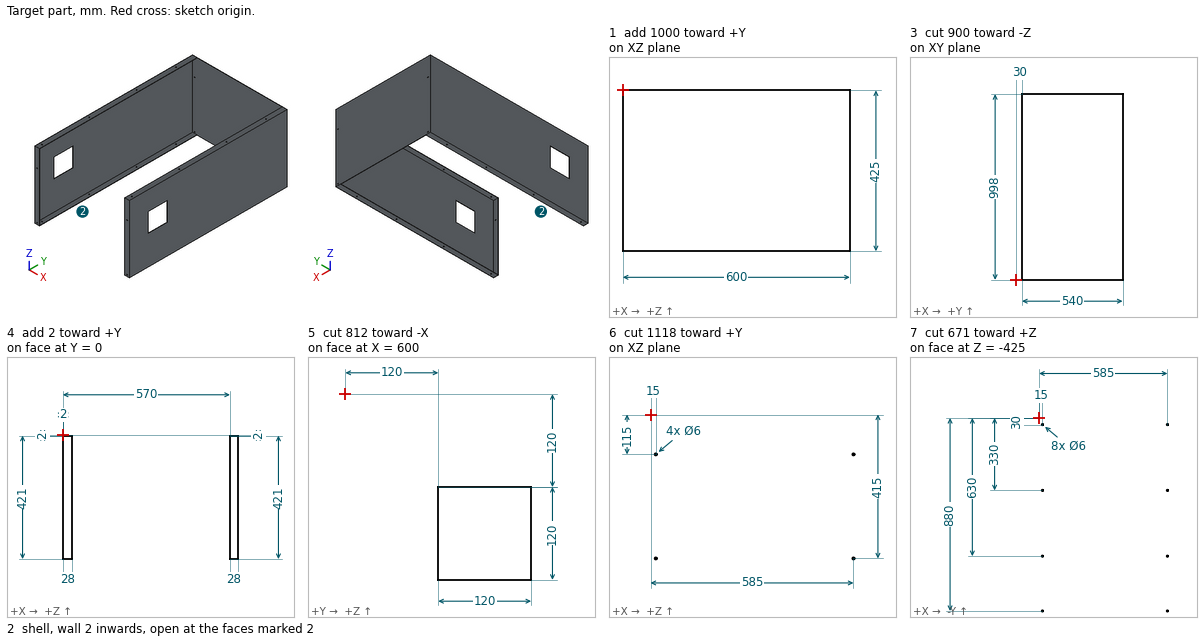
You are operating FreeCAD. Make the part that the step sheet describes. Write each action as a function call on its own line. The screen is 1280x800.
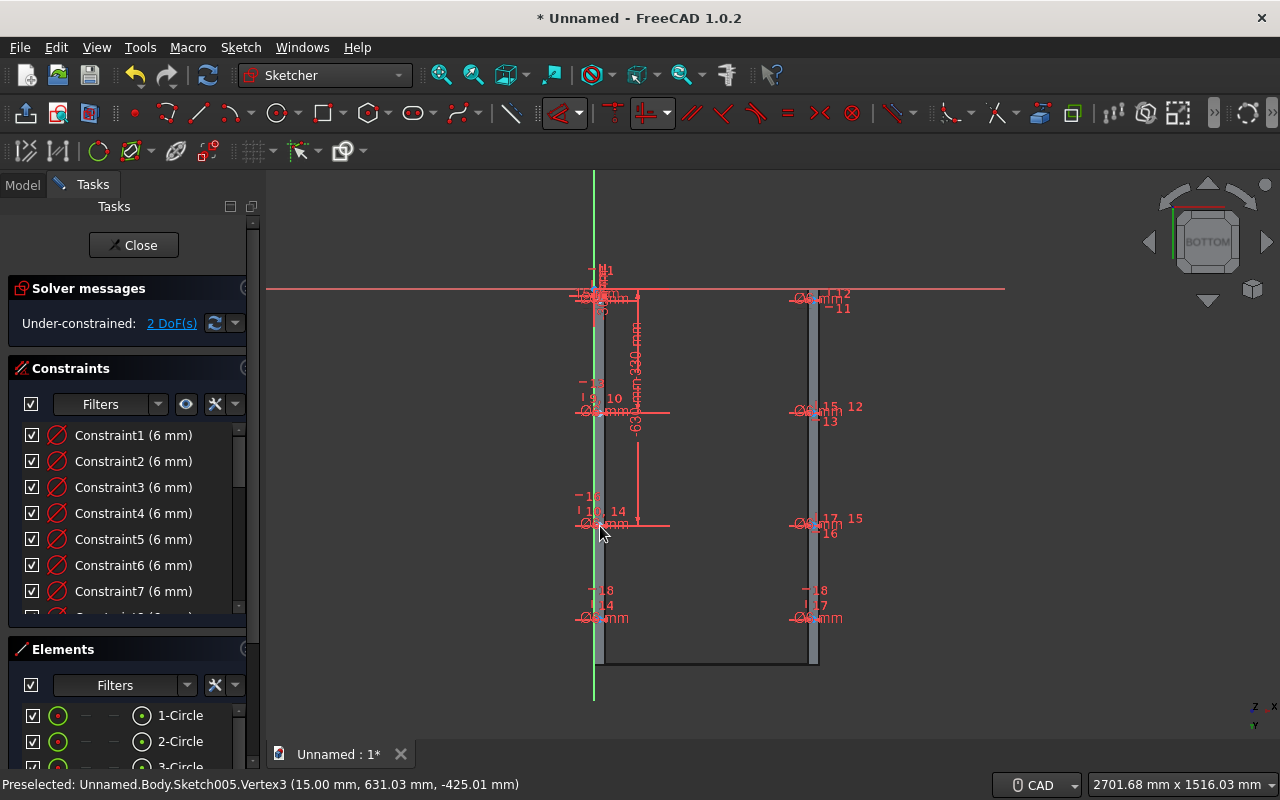
click(814, 301)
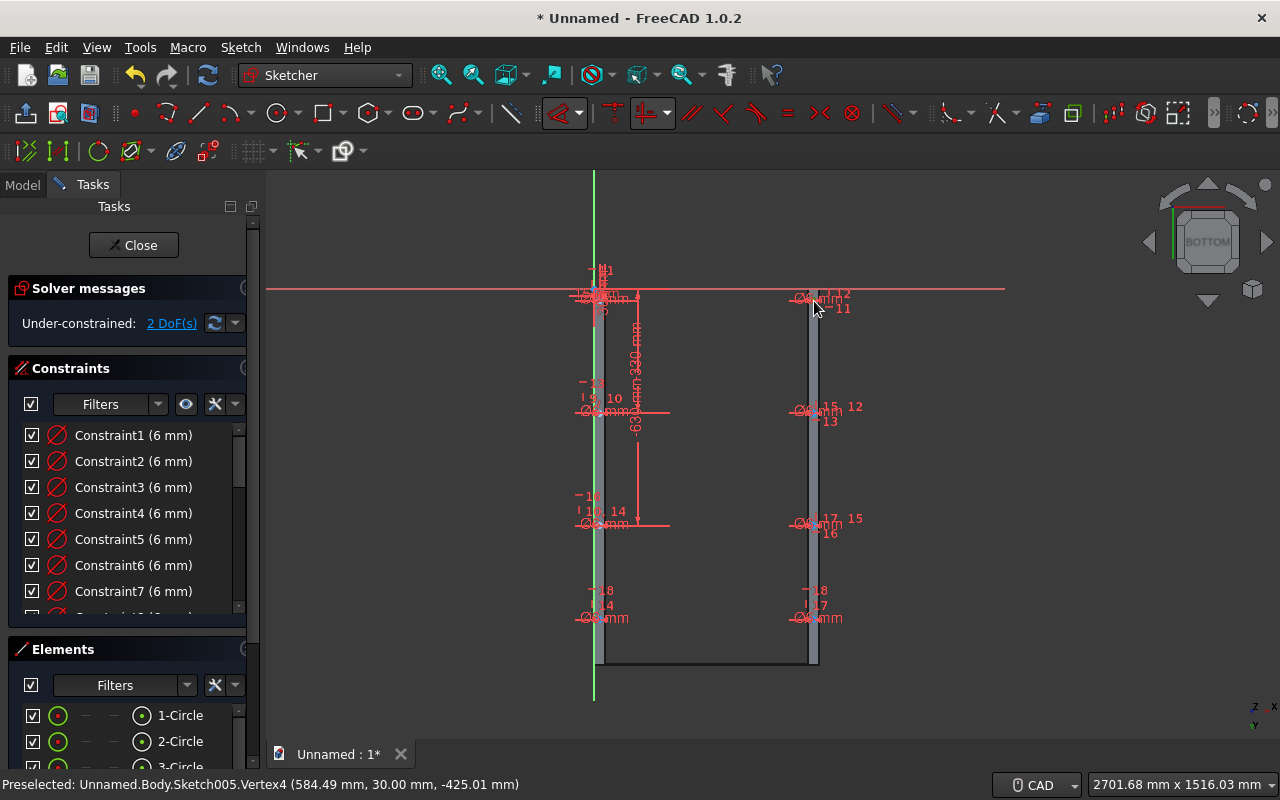
key(l)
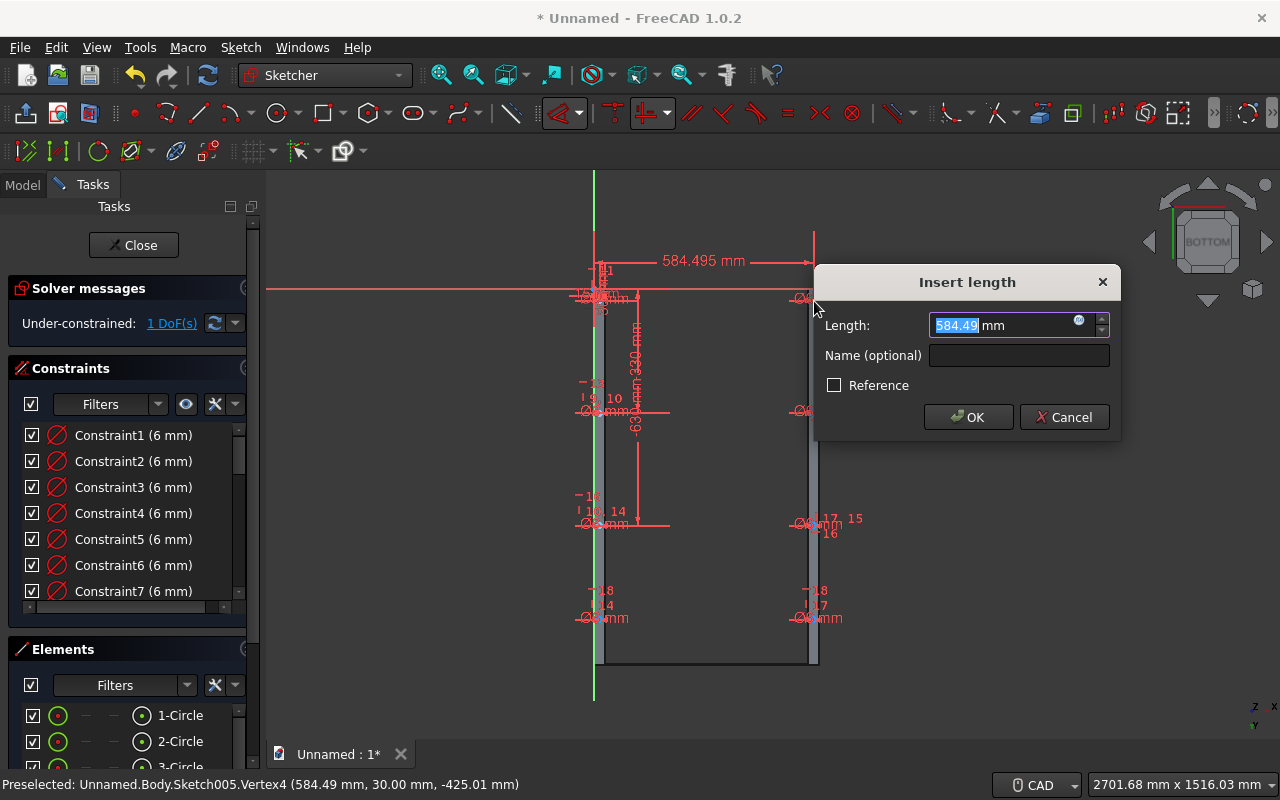
text(585)
key(Return)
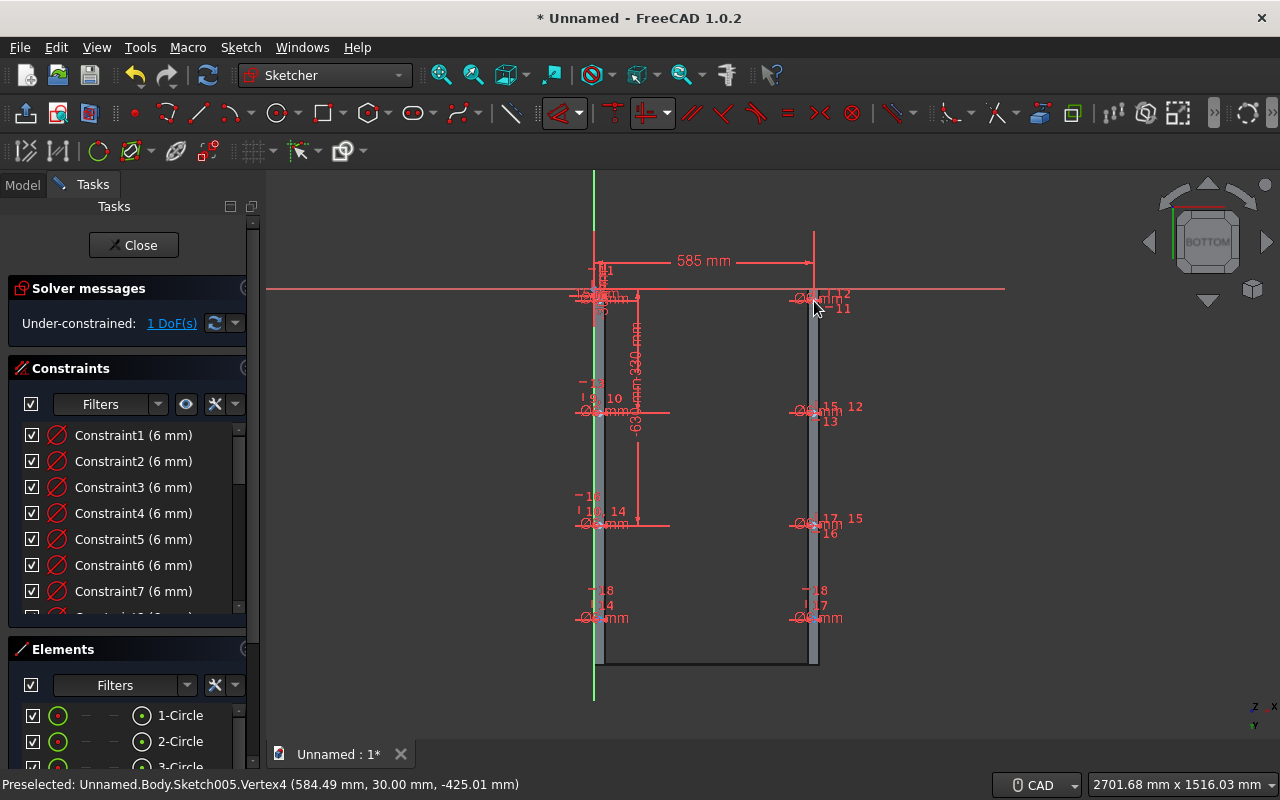
click(600, 620)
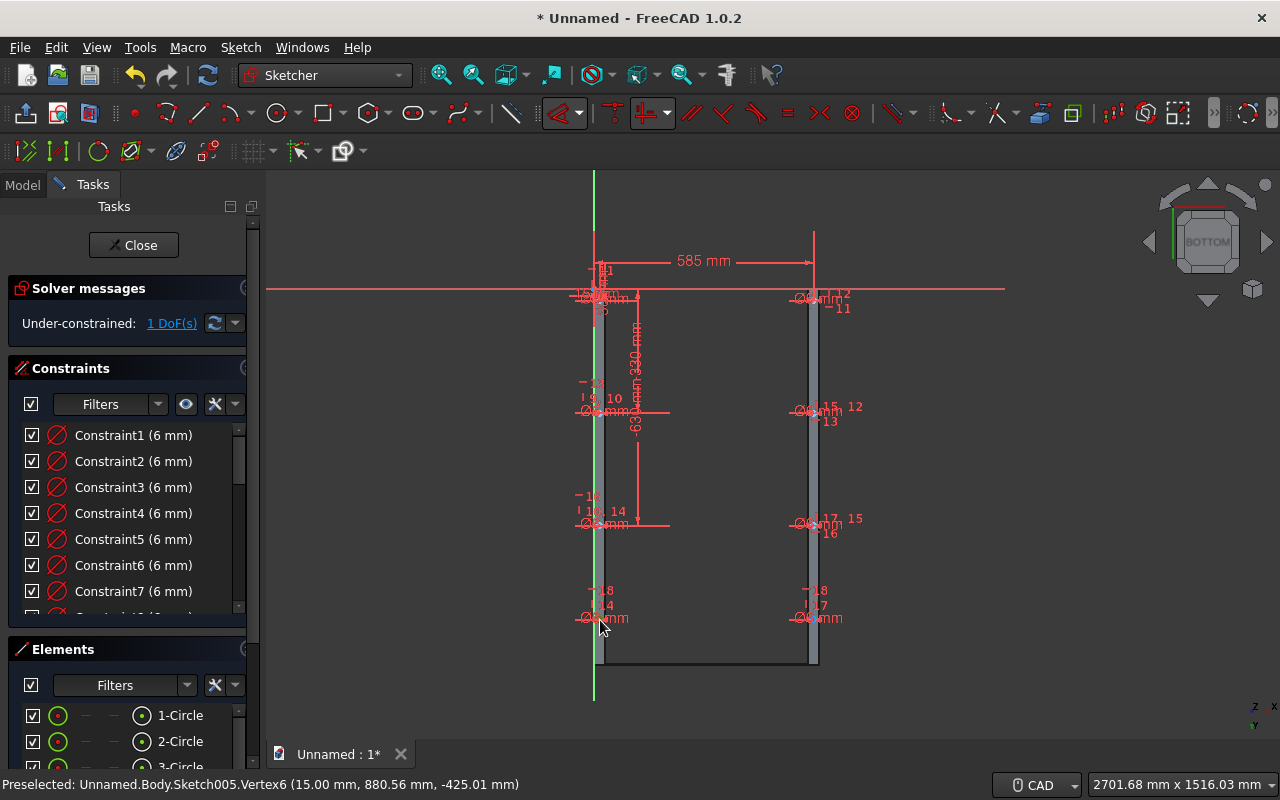
click(582, 114)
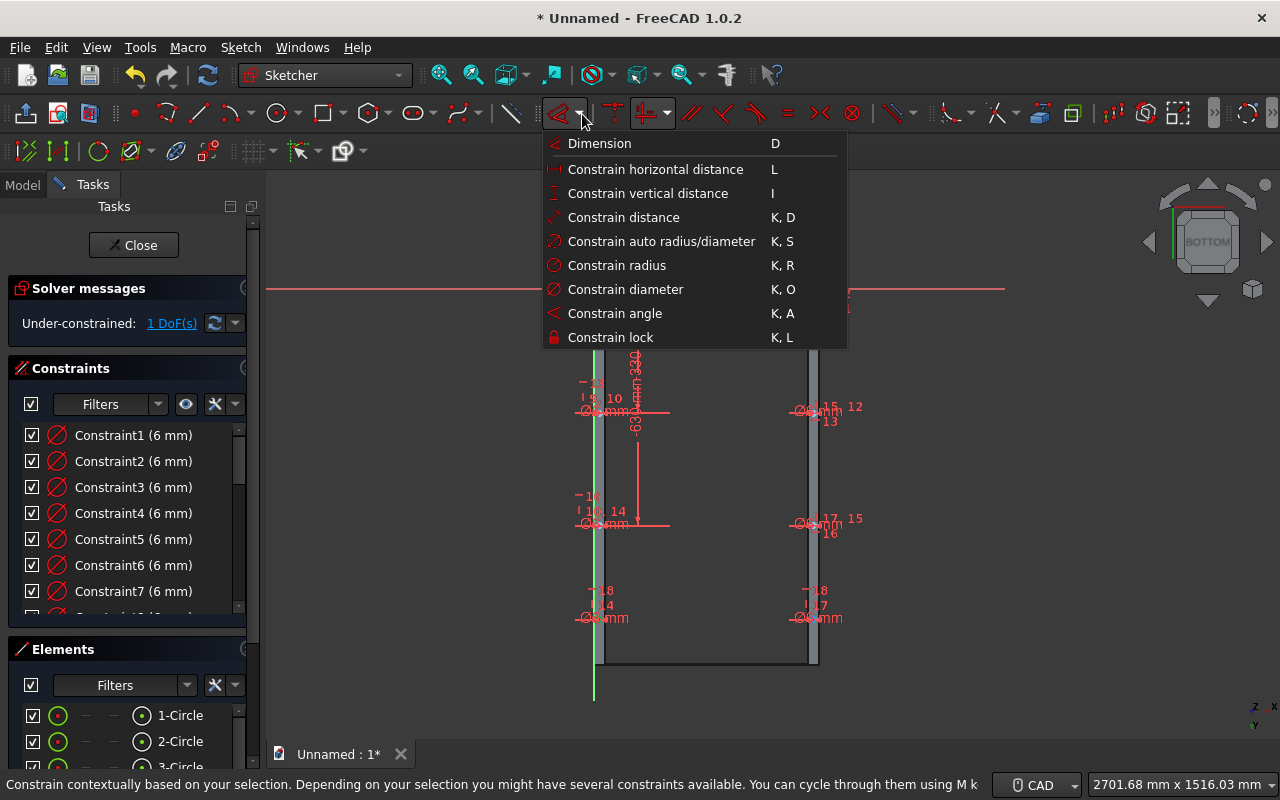
click(695, 193)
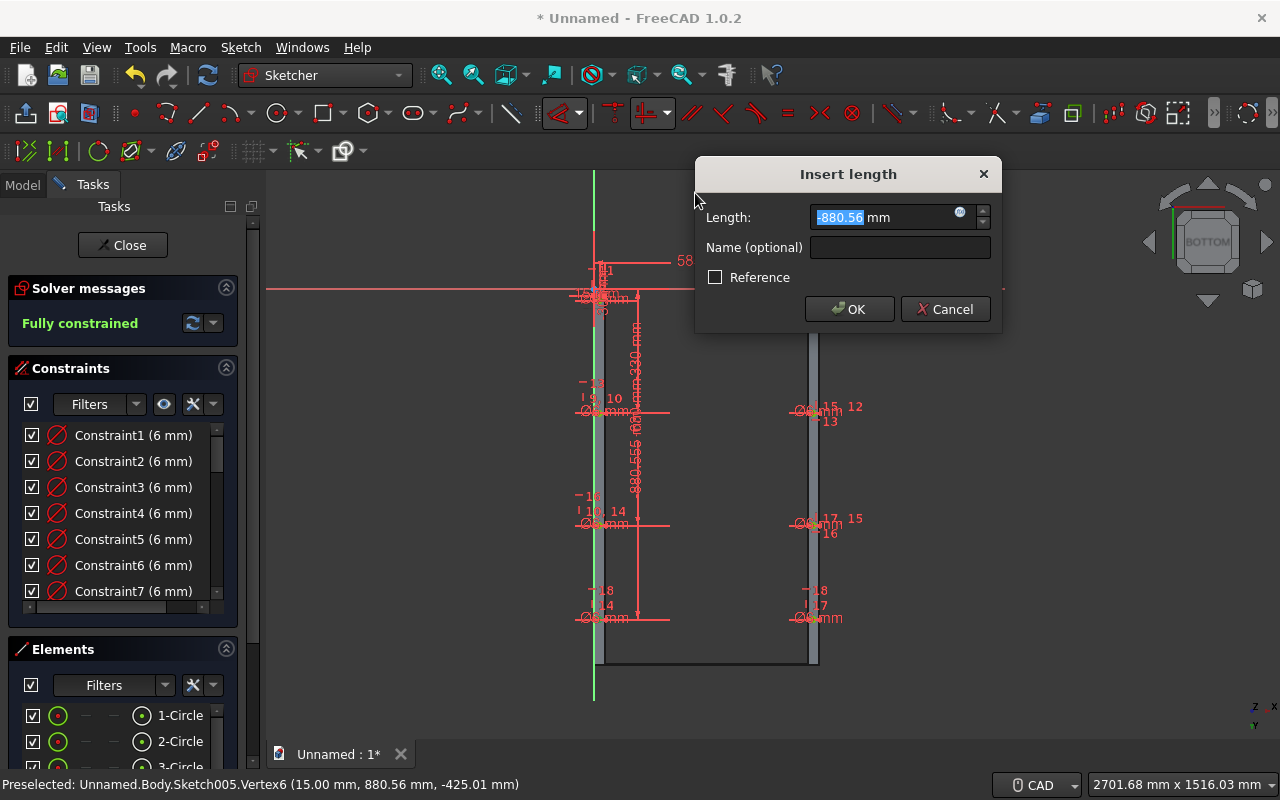
text(-880)
key(Return)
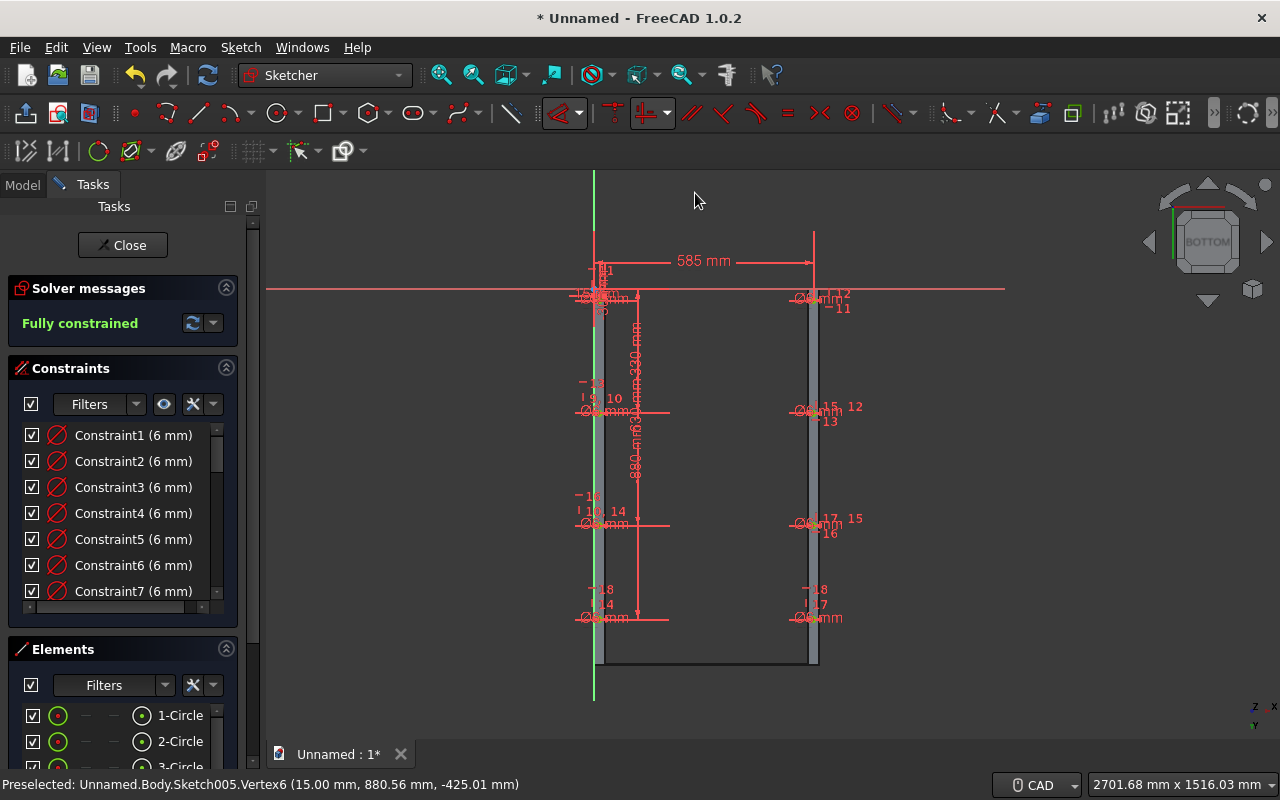
click(123, 245)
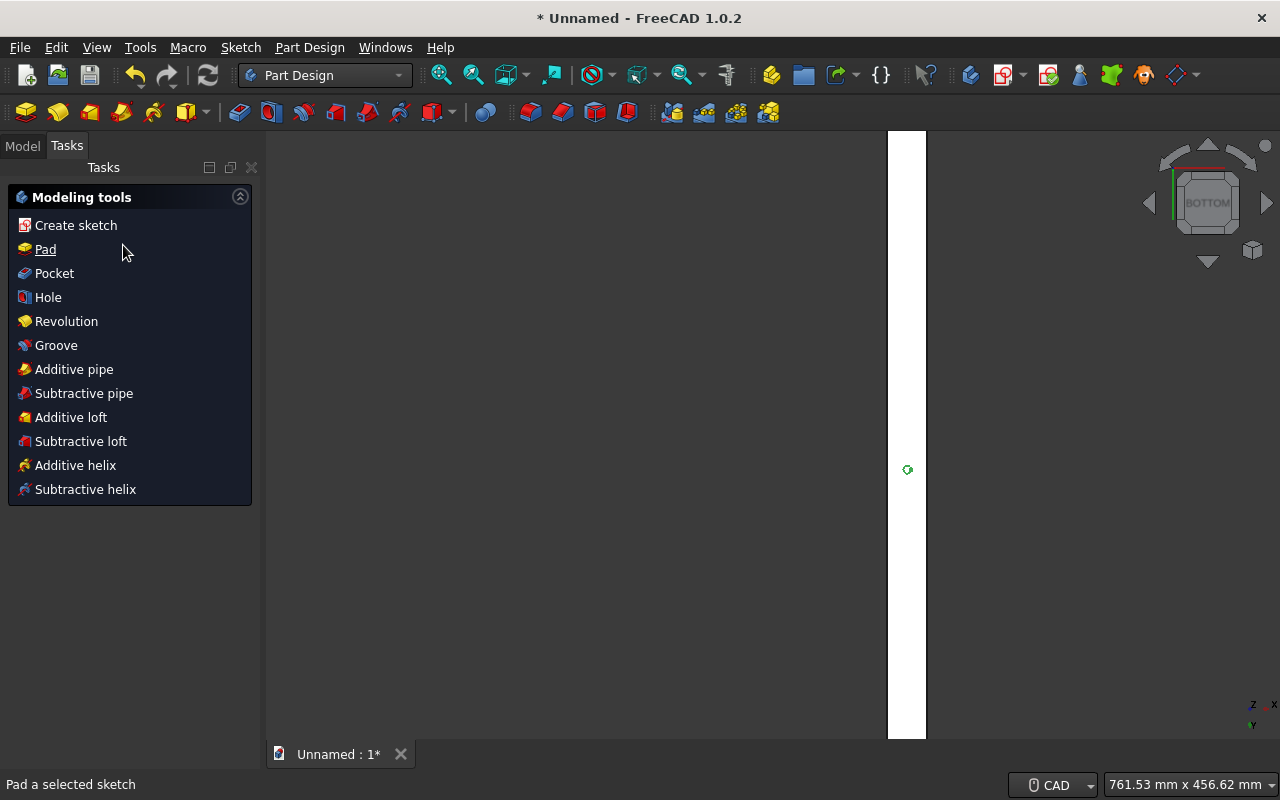
click(240, 112)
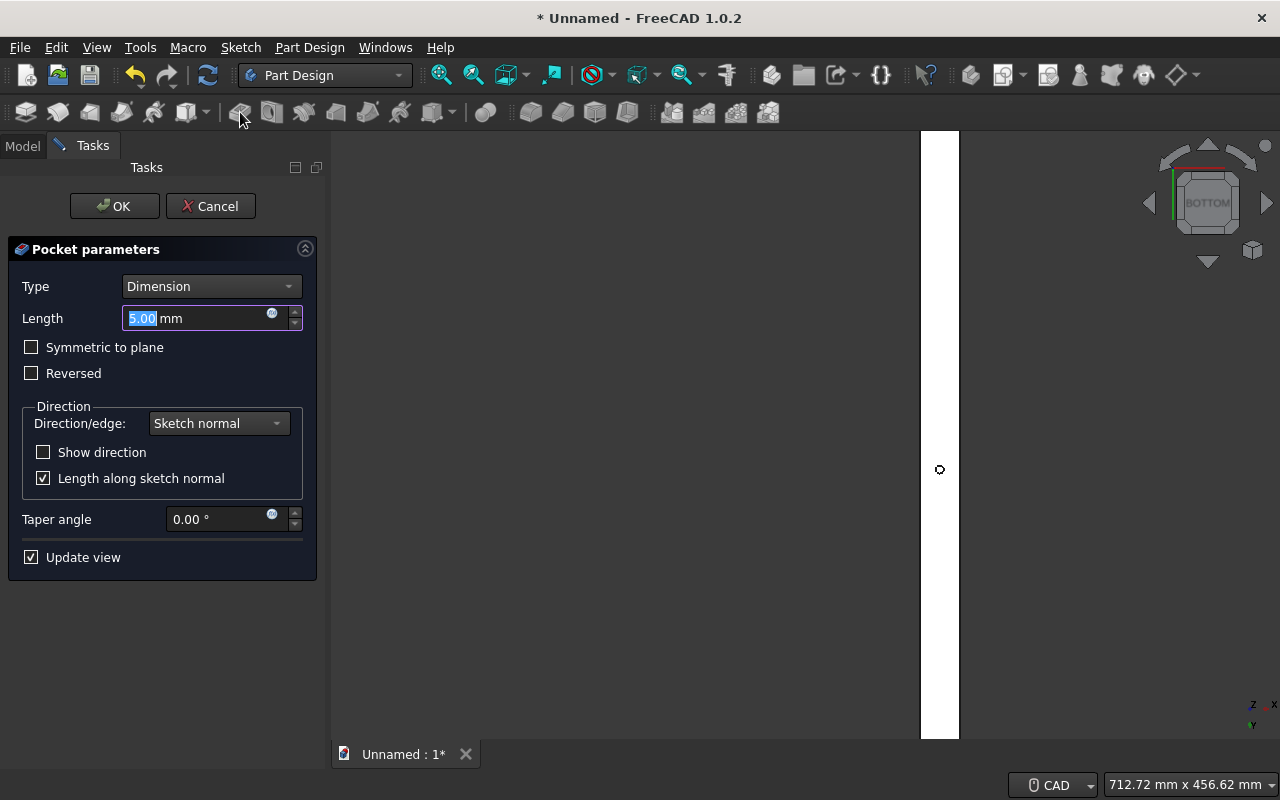
text(671)
key(Tab)